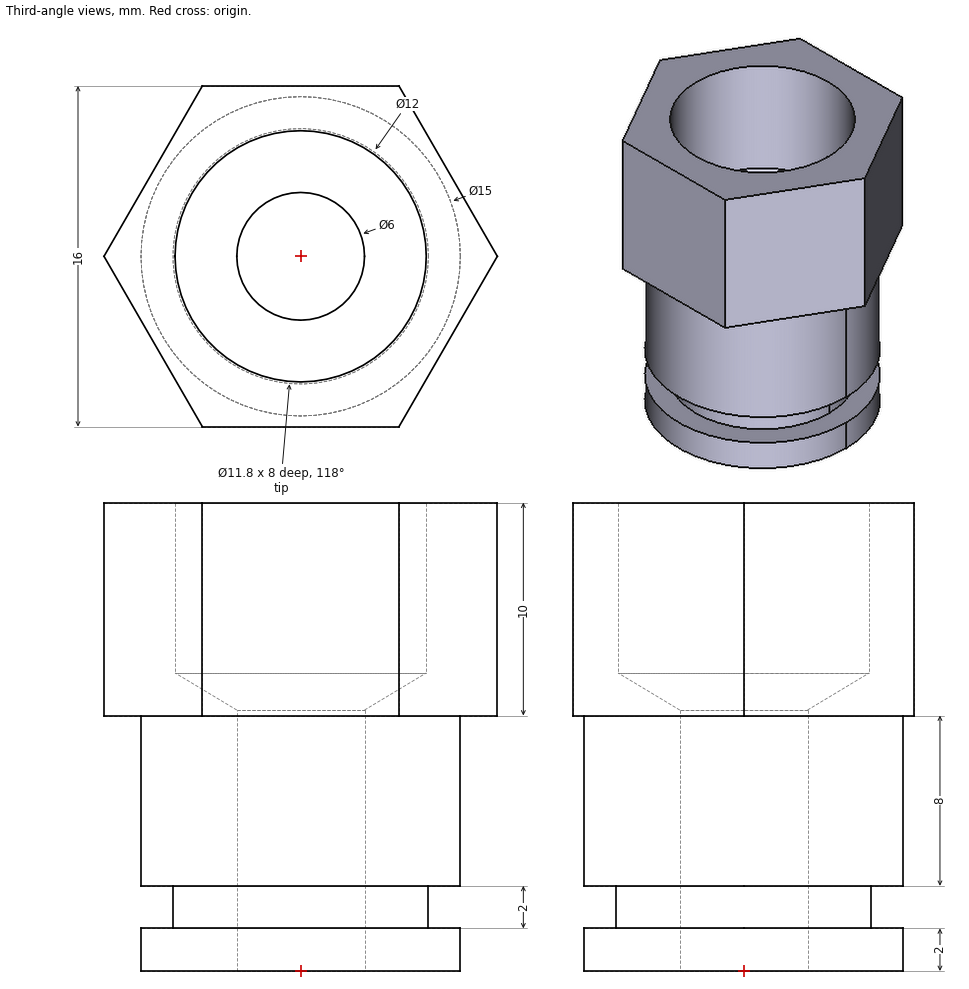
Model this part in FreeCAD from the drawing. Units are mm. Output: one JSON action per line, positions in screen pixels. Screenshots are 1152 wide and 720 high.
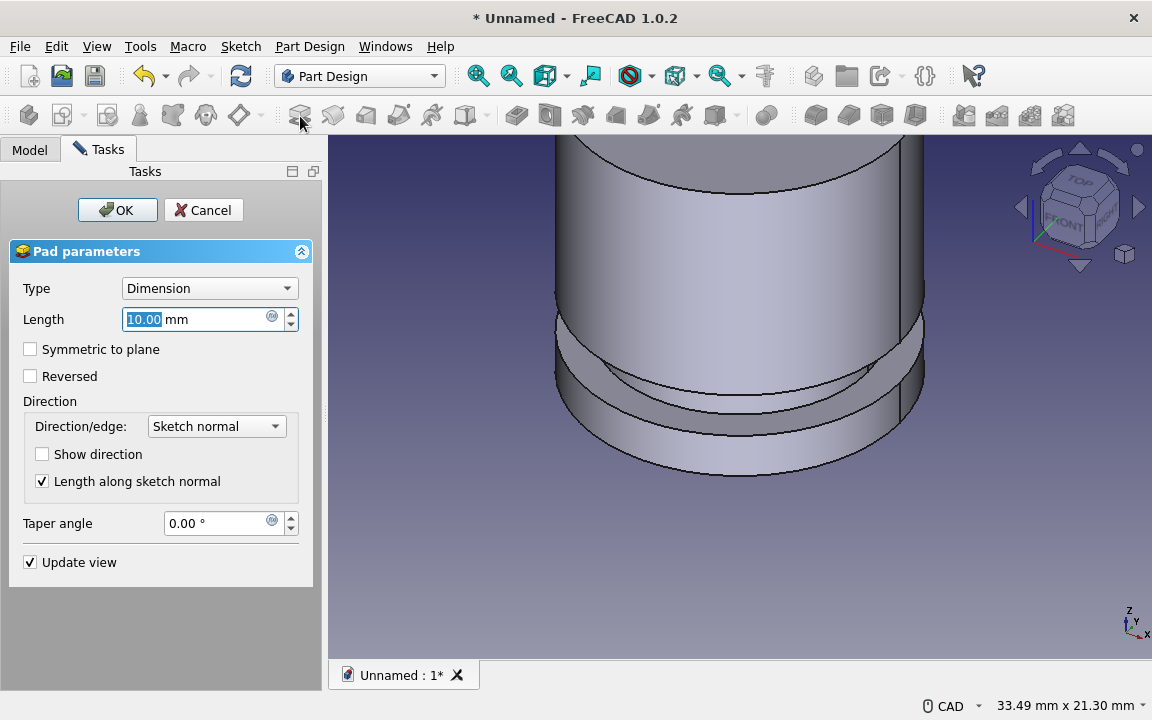
{"action": "type", "text": "8"}
{"action": "key", "text": "Tab"}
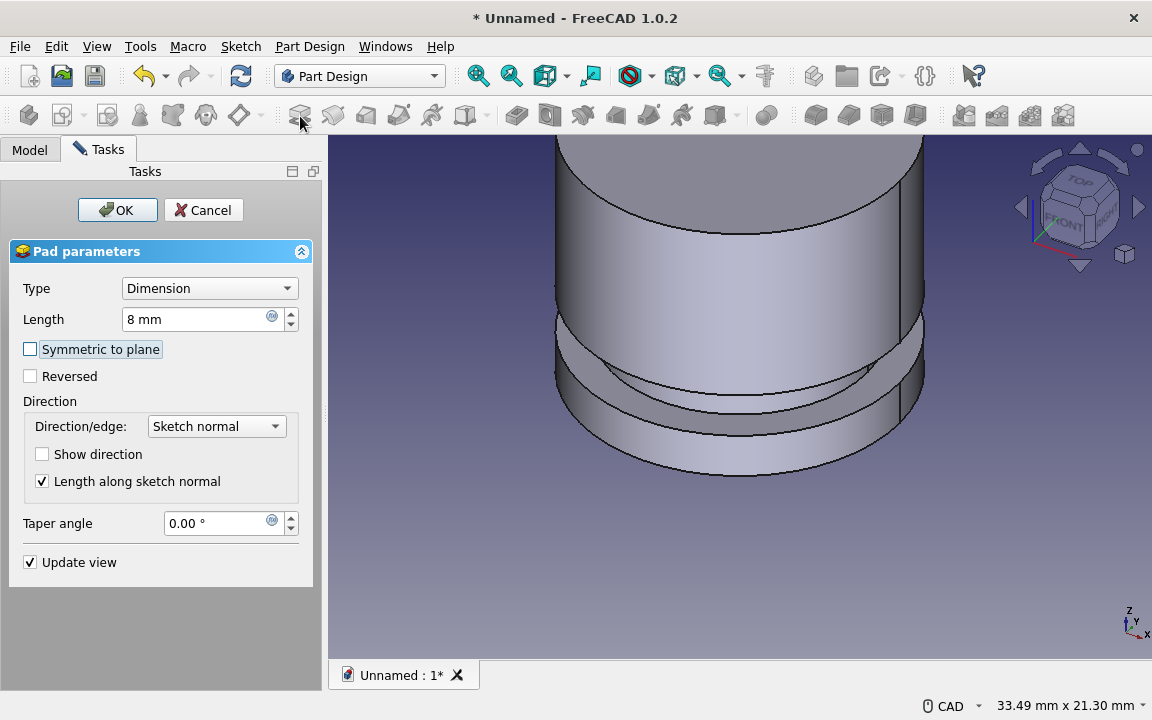
{"action": "left_click", "coordinate": [118, 210]}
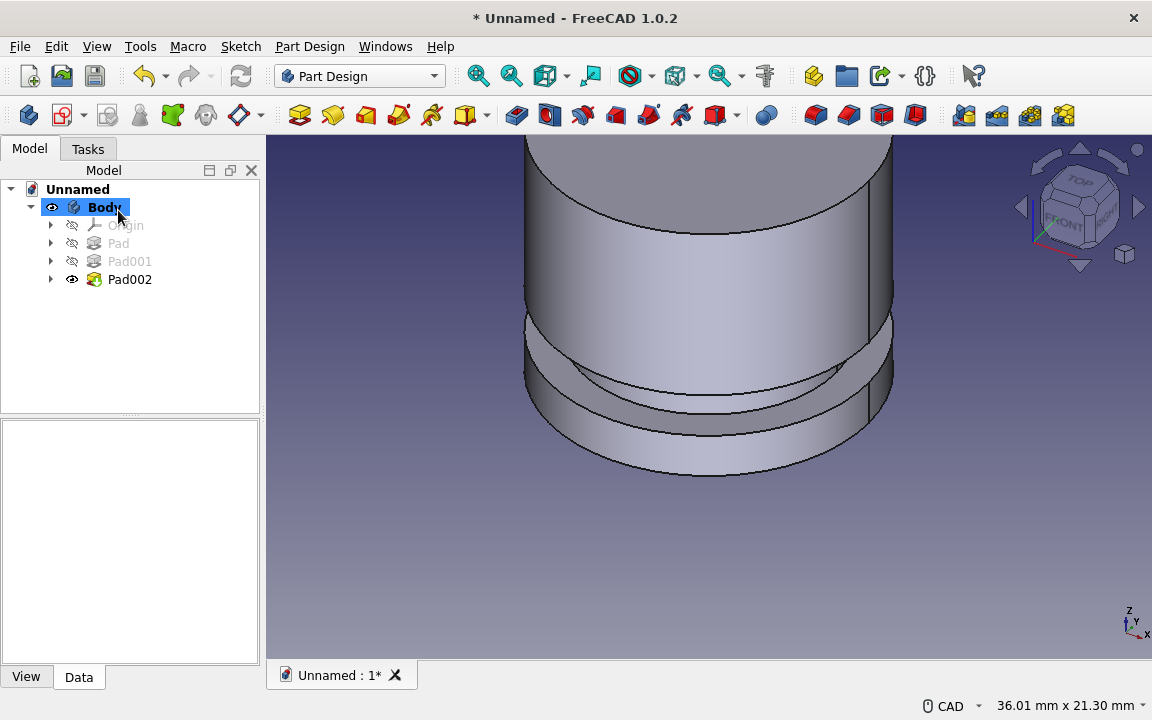
{"action": "left_click", "coordinate": [479, 76]}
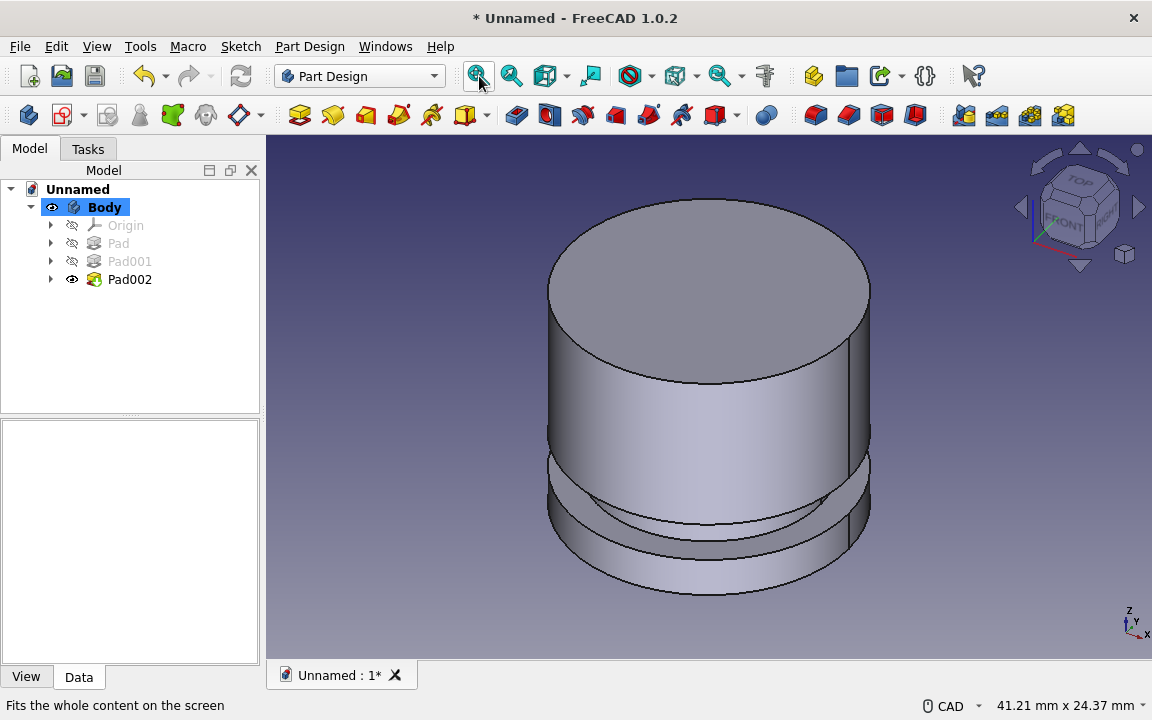
{"action": "left_click", "coordinate": [709, 290]}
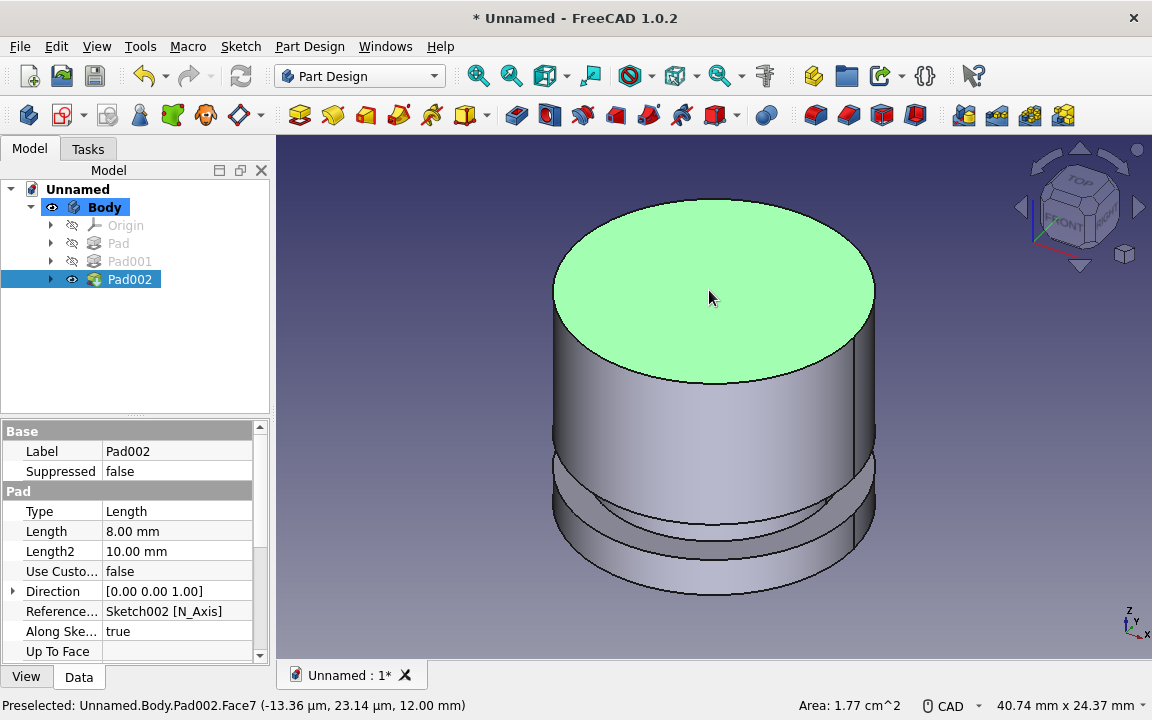
{"action": "left_click", "coordinate": [62, 116]}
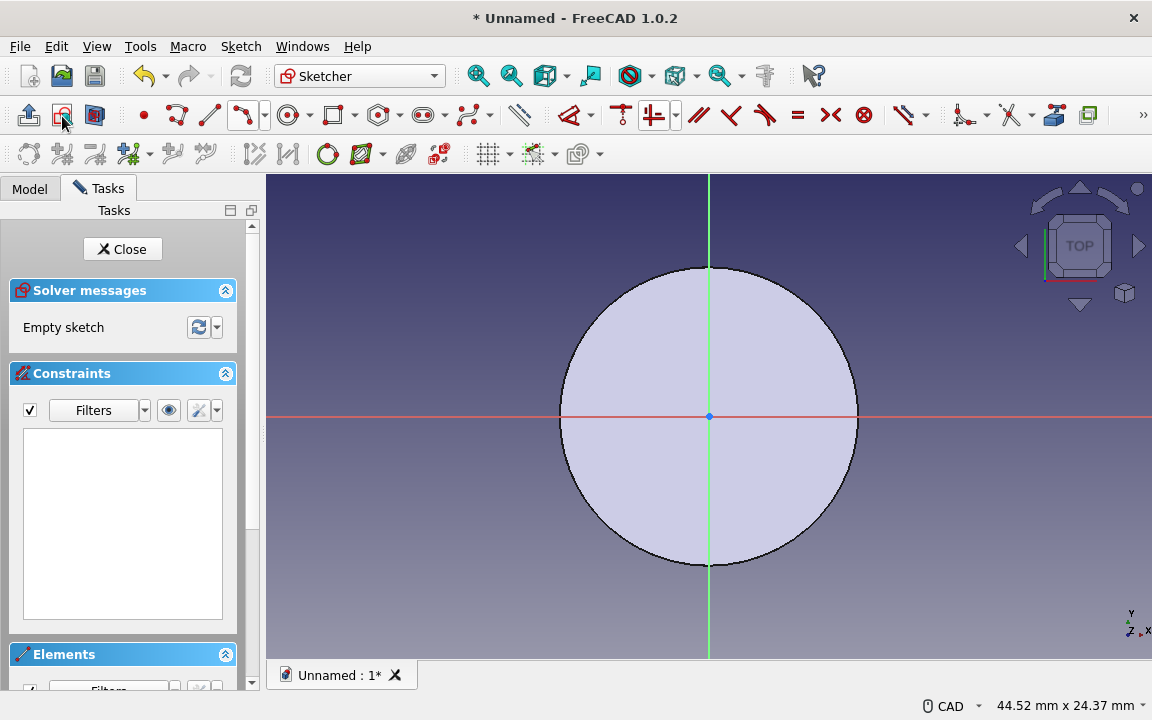
{"action": "key", "text": "g p 6"}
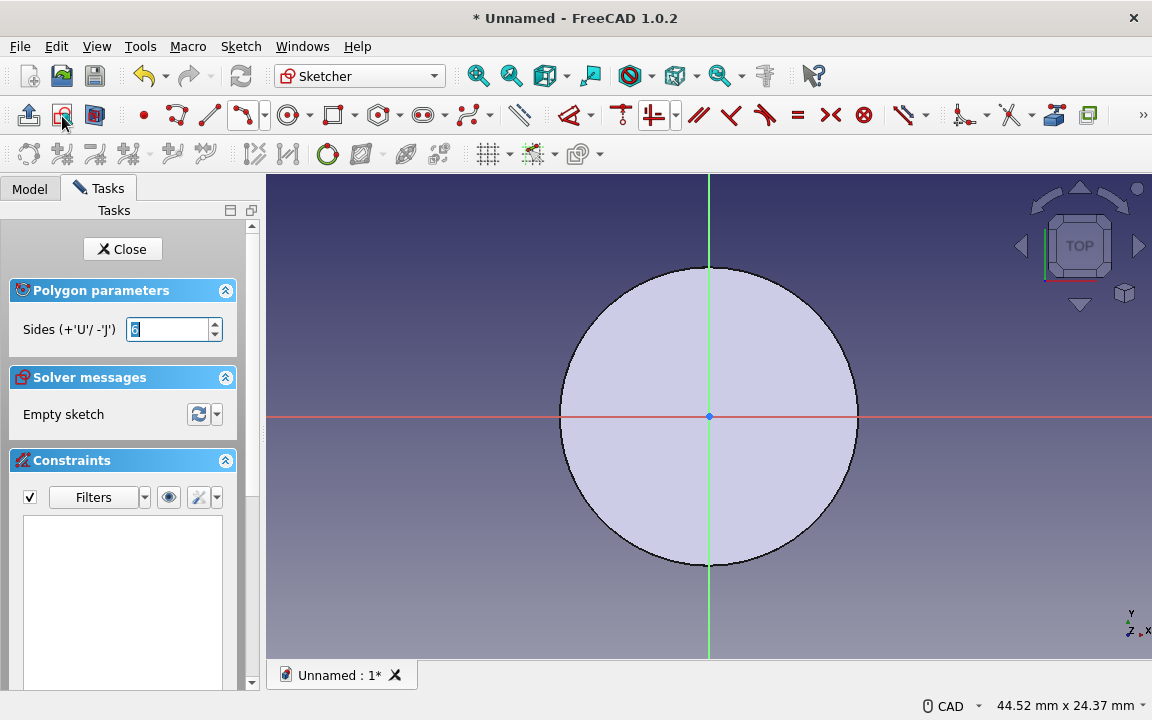
{"action": "left_click", "coordinate": [709, 416]}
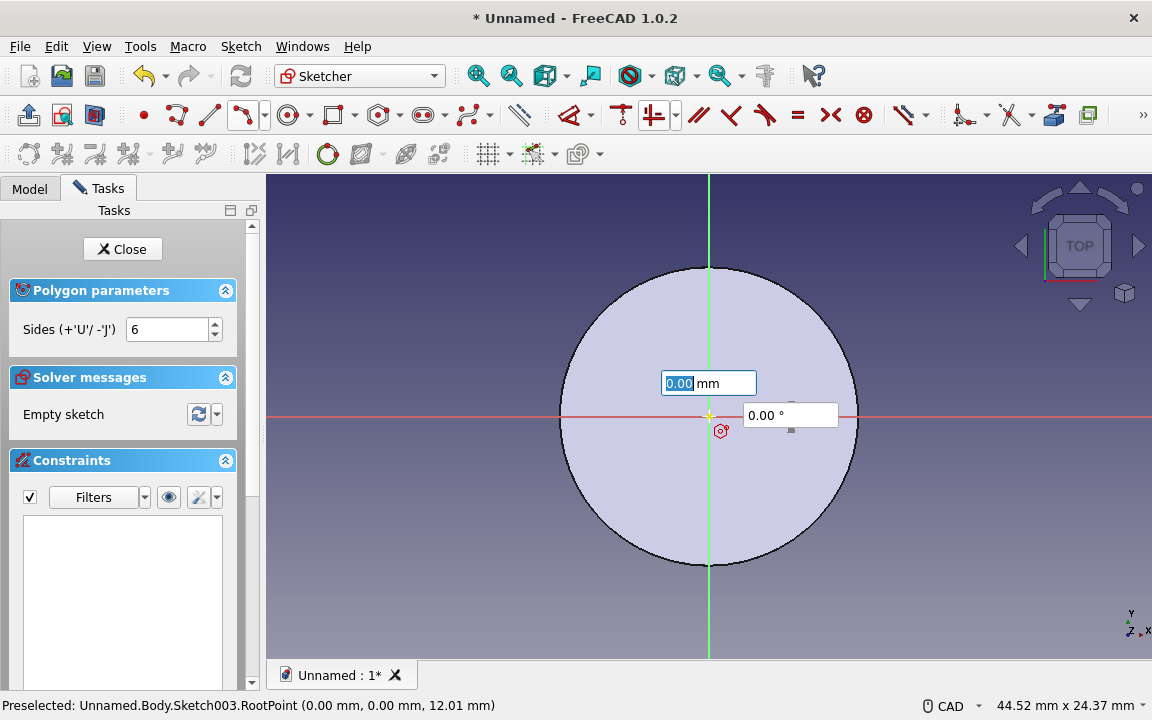
{"action": "left_click", "coordinate": [893, 416]}
{"action": "right_click", "coordinate": [893, 416]}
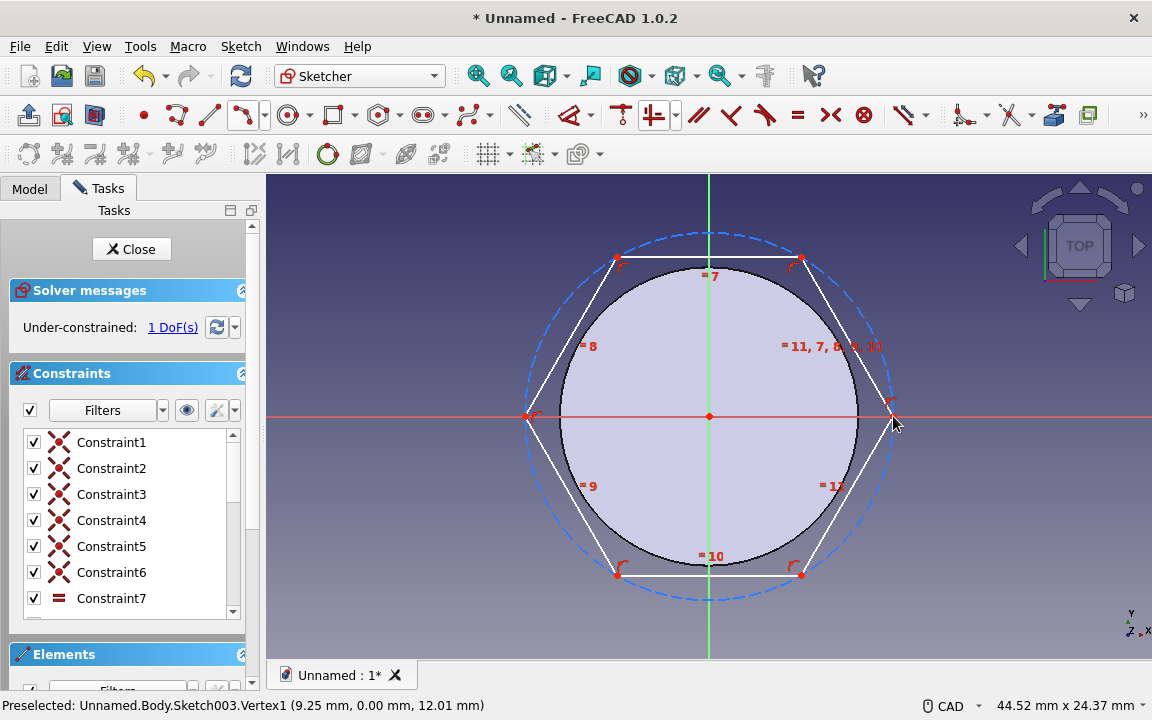
{"action": "left_click", "coordinate": [568, 116]}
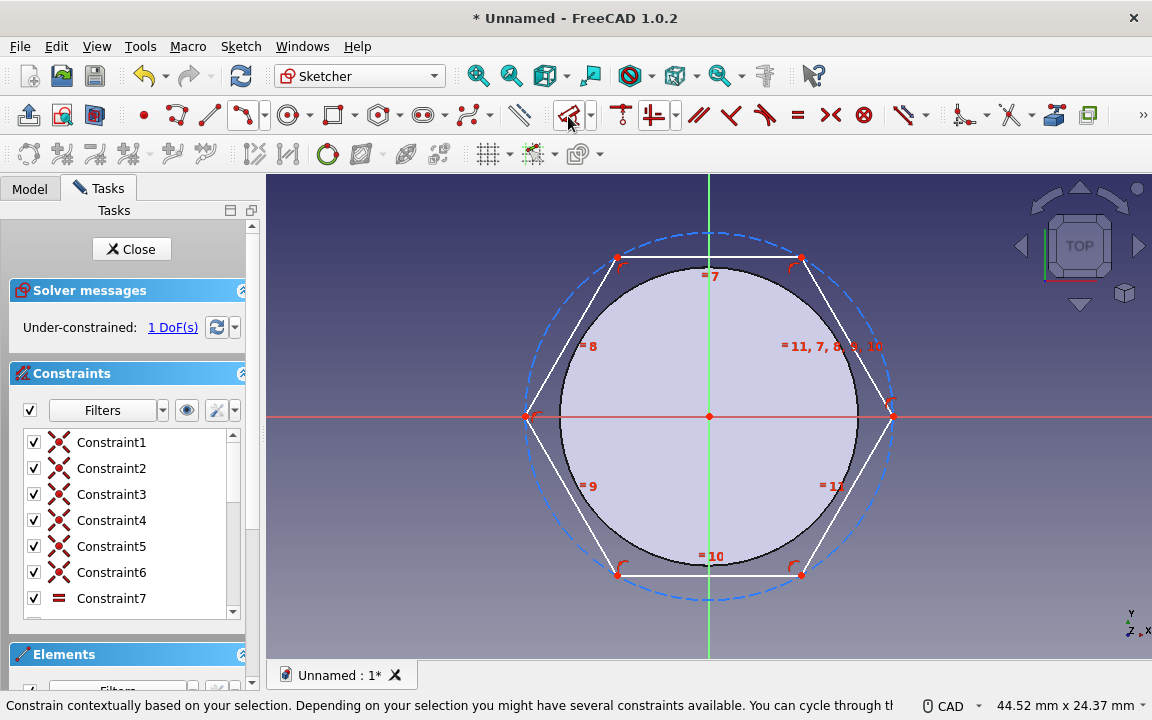
{"action": "left_click", "coordinate": [617, 576]}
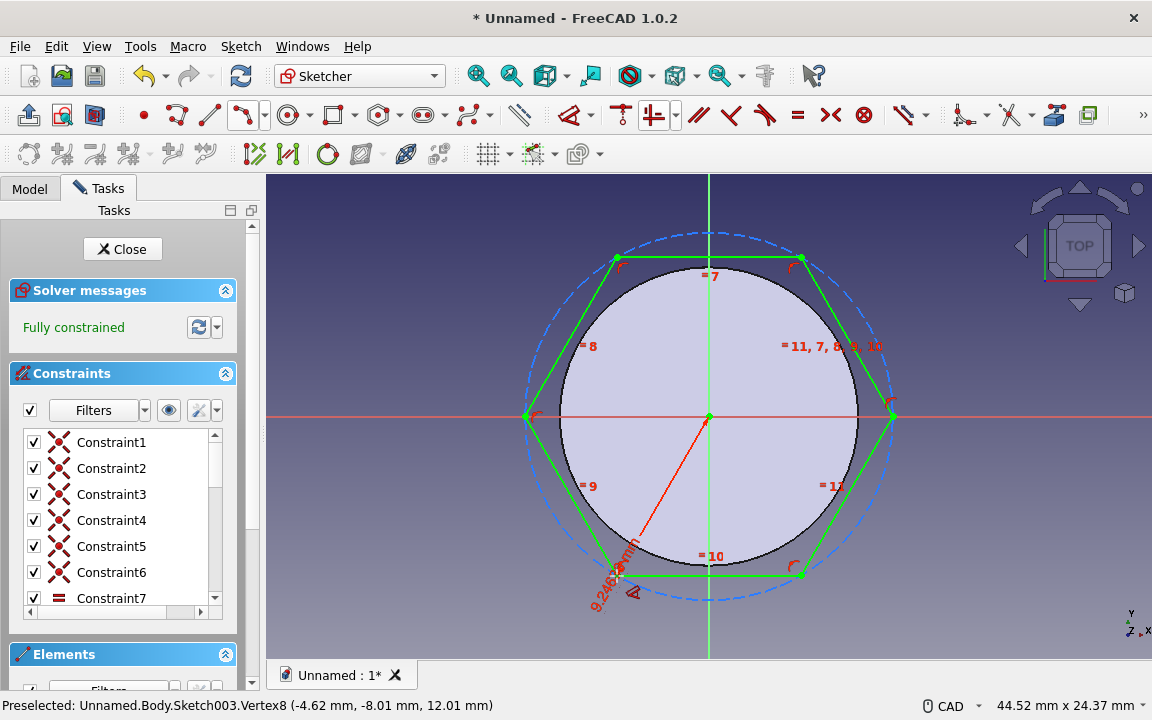
{"action": "left_click", "coordinate": [801, 257]}
{"action": "left_click", "coordinate": [835, 343]}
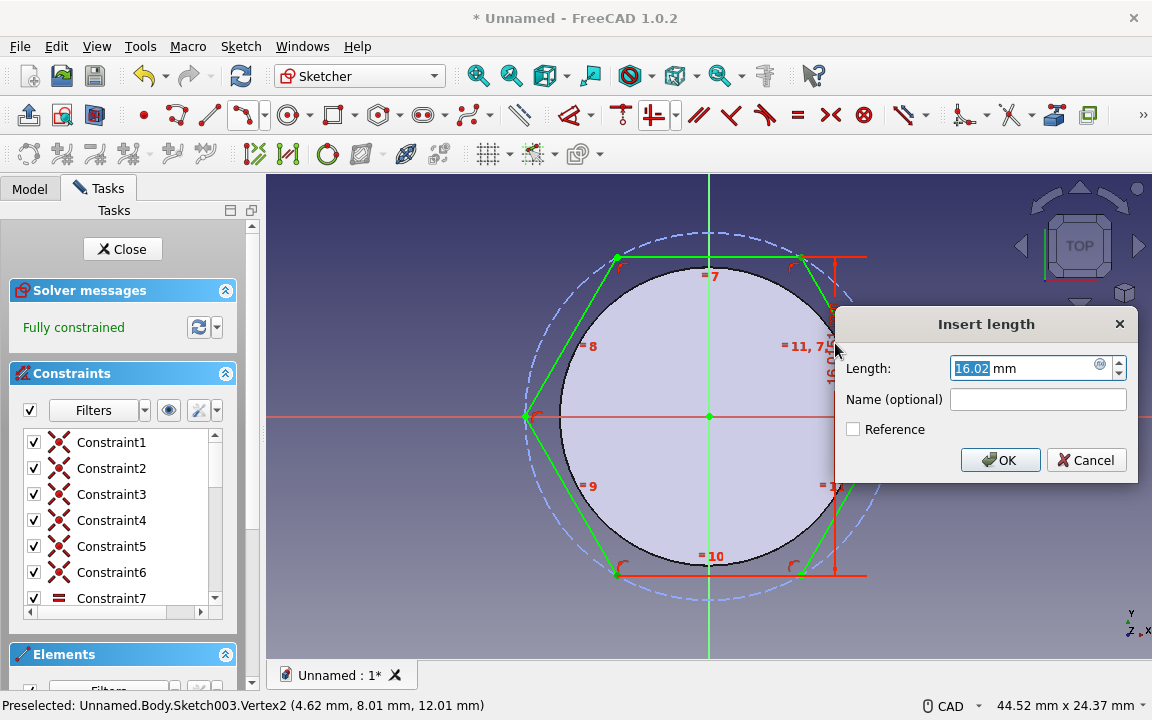
{"action": "type", "text": "16"}
{"action": "key", "text": "Return"}
{"action": "key", "text": "Escape"}